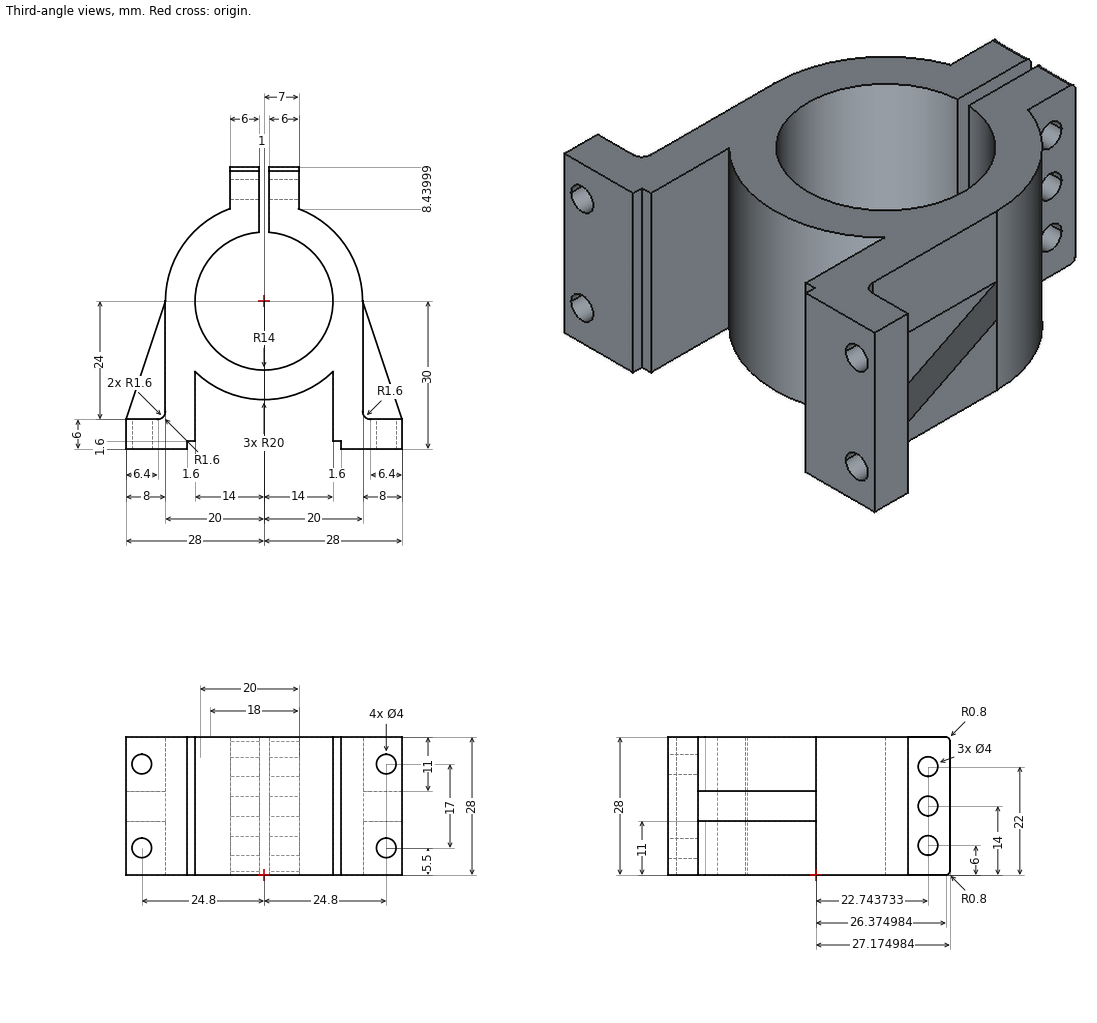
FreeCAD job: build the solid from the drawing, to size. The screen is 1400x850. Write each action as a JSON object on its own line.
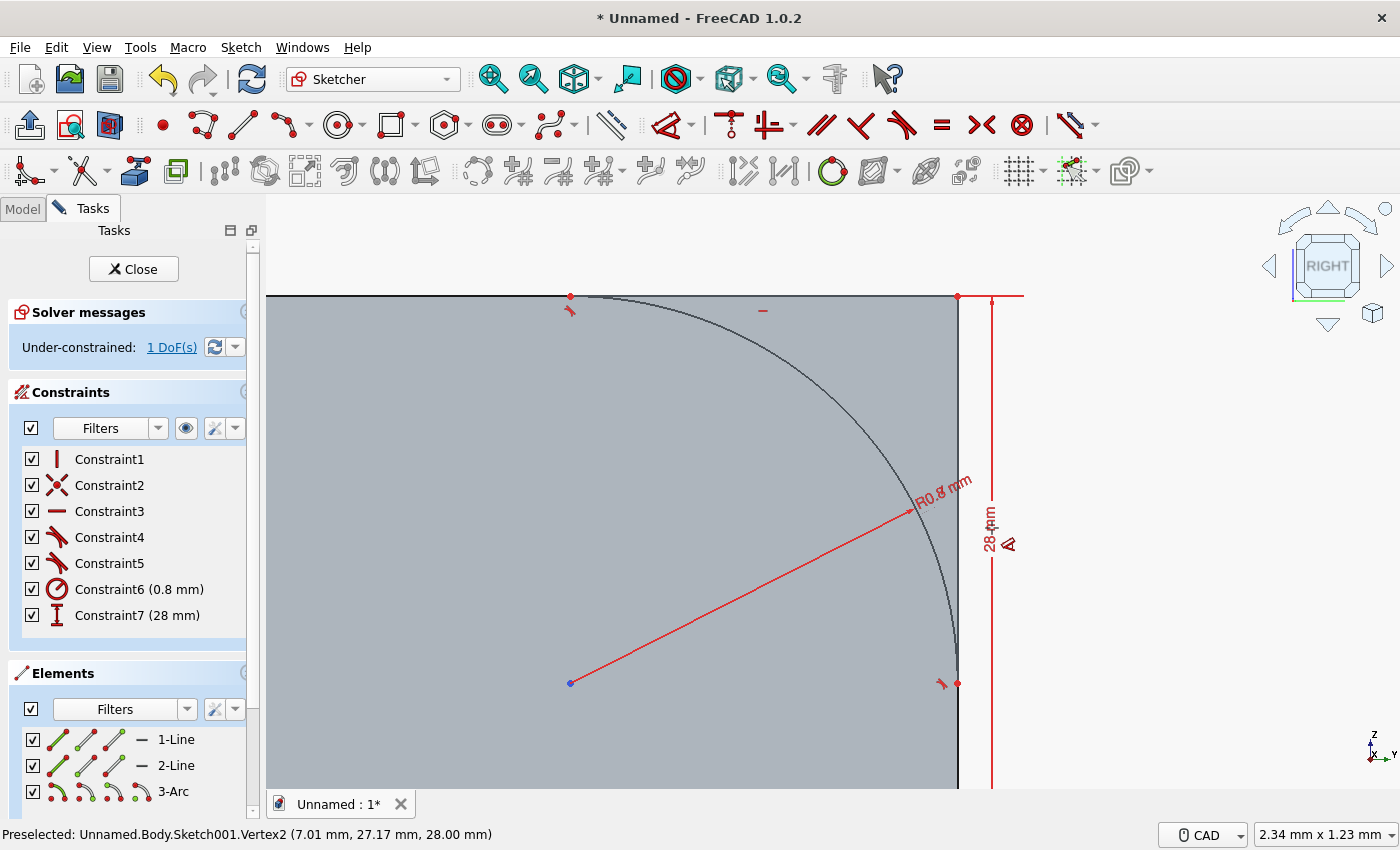
{"action": "left_click", "coordinate": [958, 684]}
{"action": "left_click", "coordinate": [626, 650]}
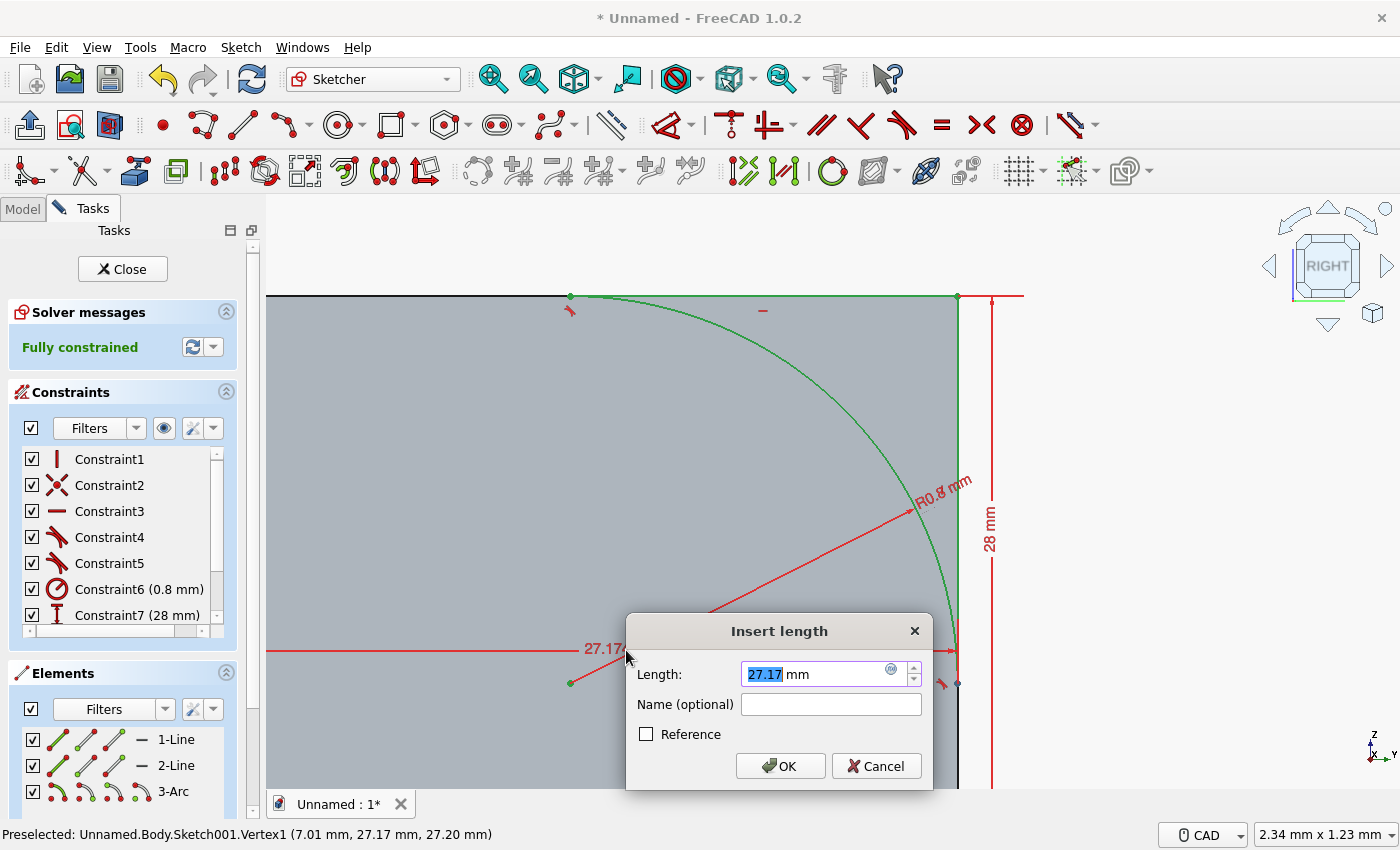
{"action": "type", "text": "27.174984"}
{"action": "key", "text": "Return"}
{"action": "key", "text": "Escape"}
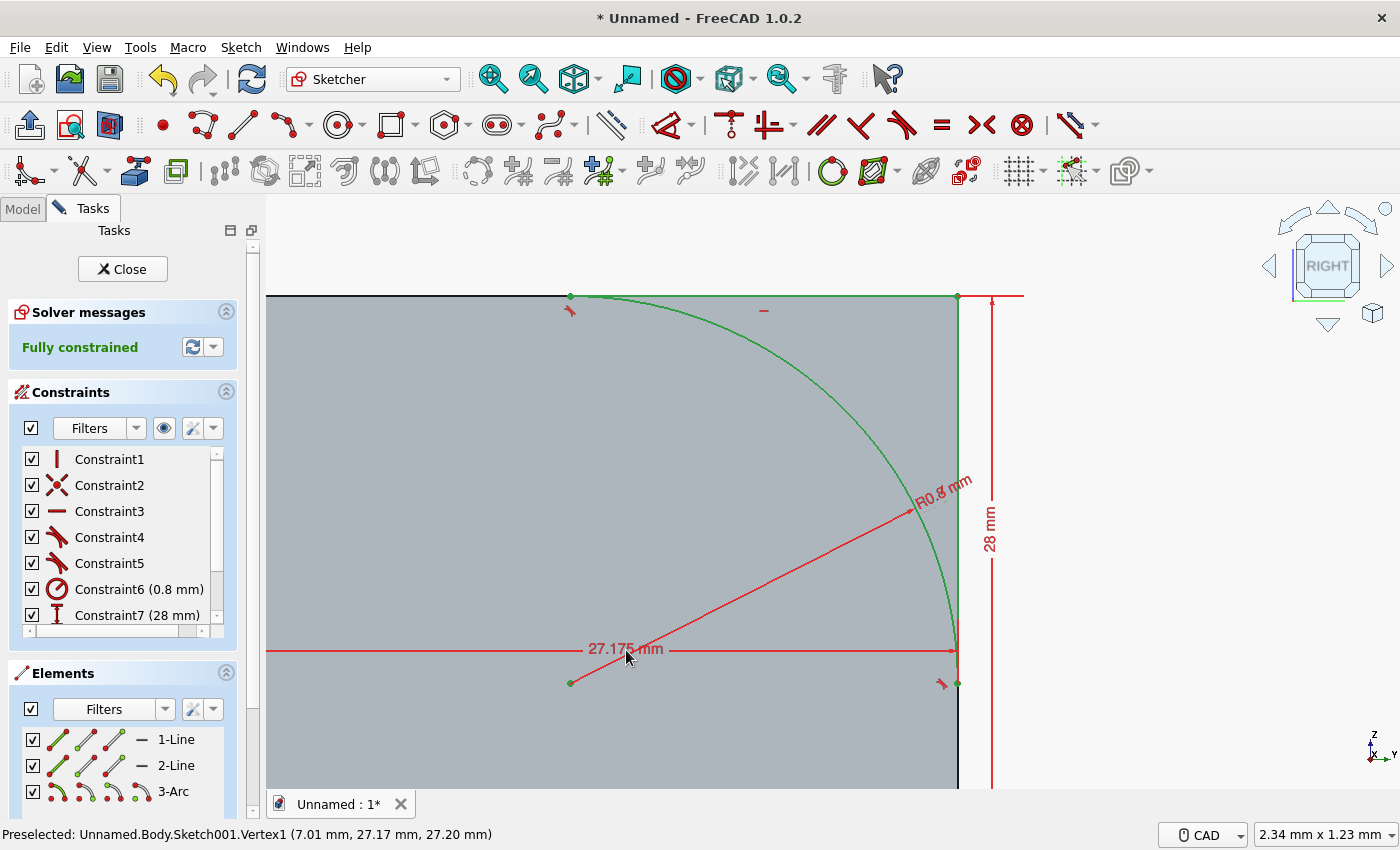
{"action": "left_click", "coordinate": [123, 269]}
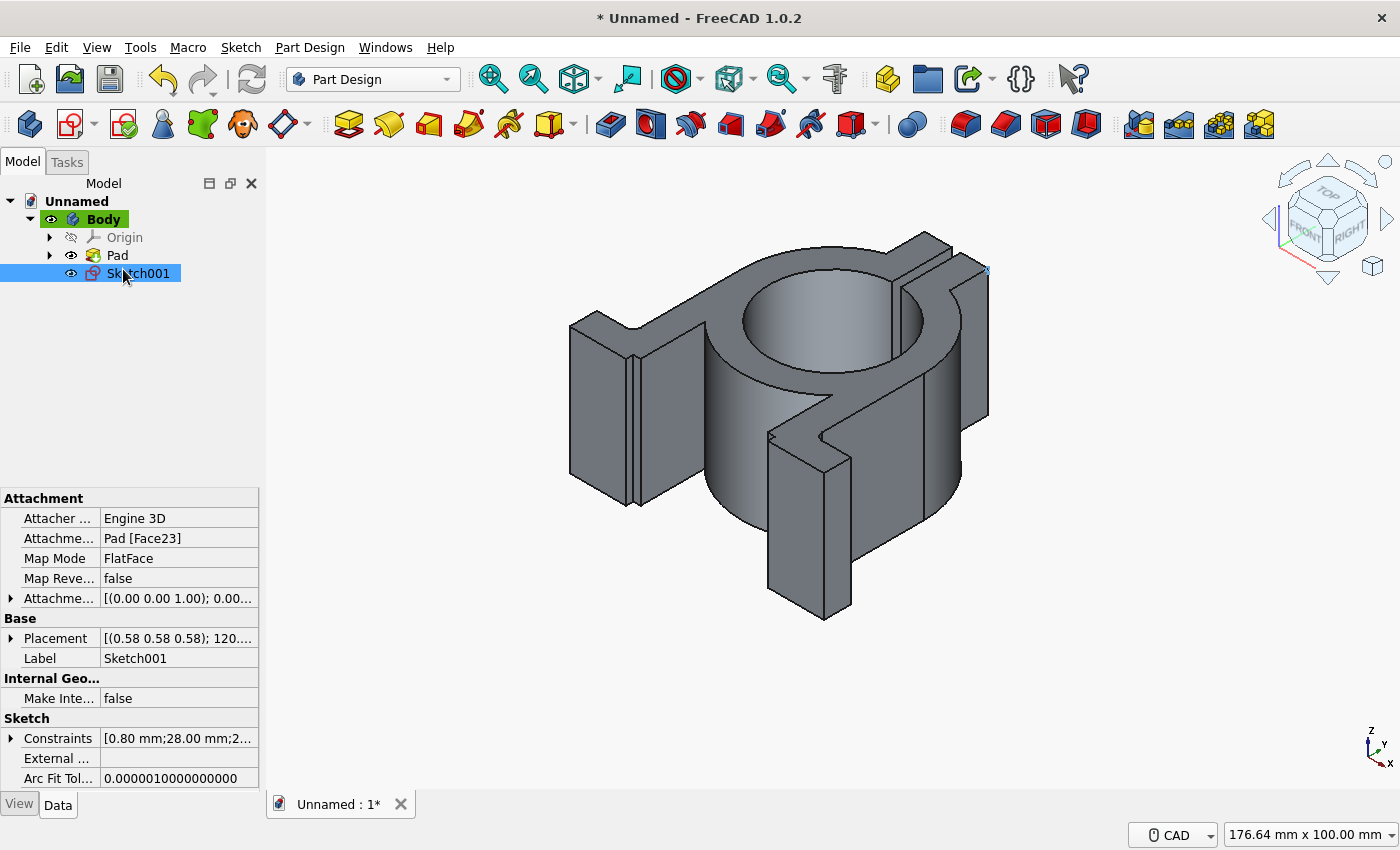
{"action": "left_click", "coordinate": [612, 124]}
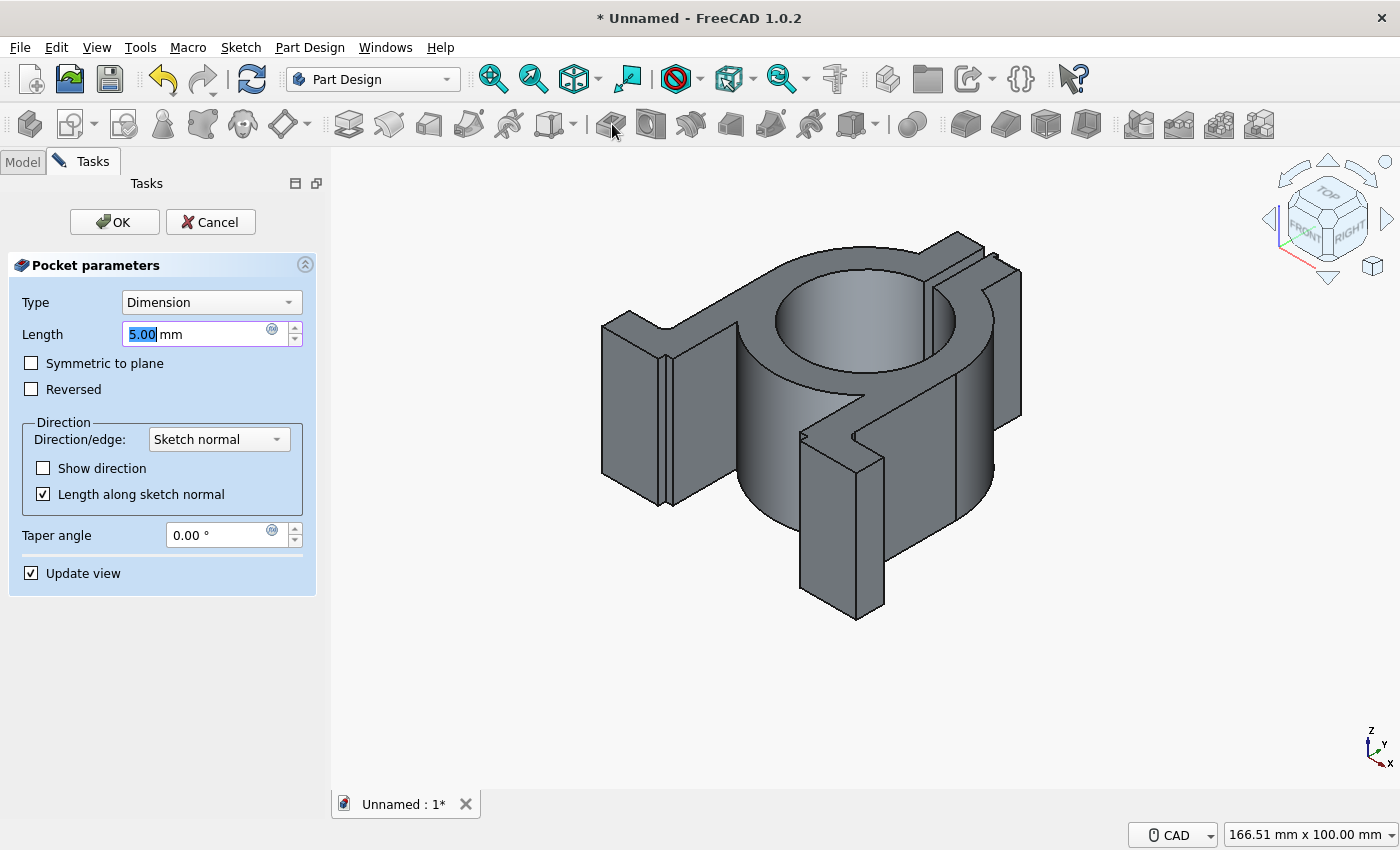
{"action": "type", "text": "18"}
{"action": "key", "text": "Tab"}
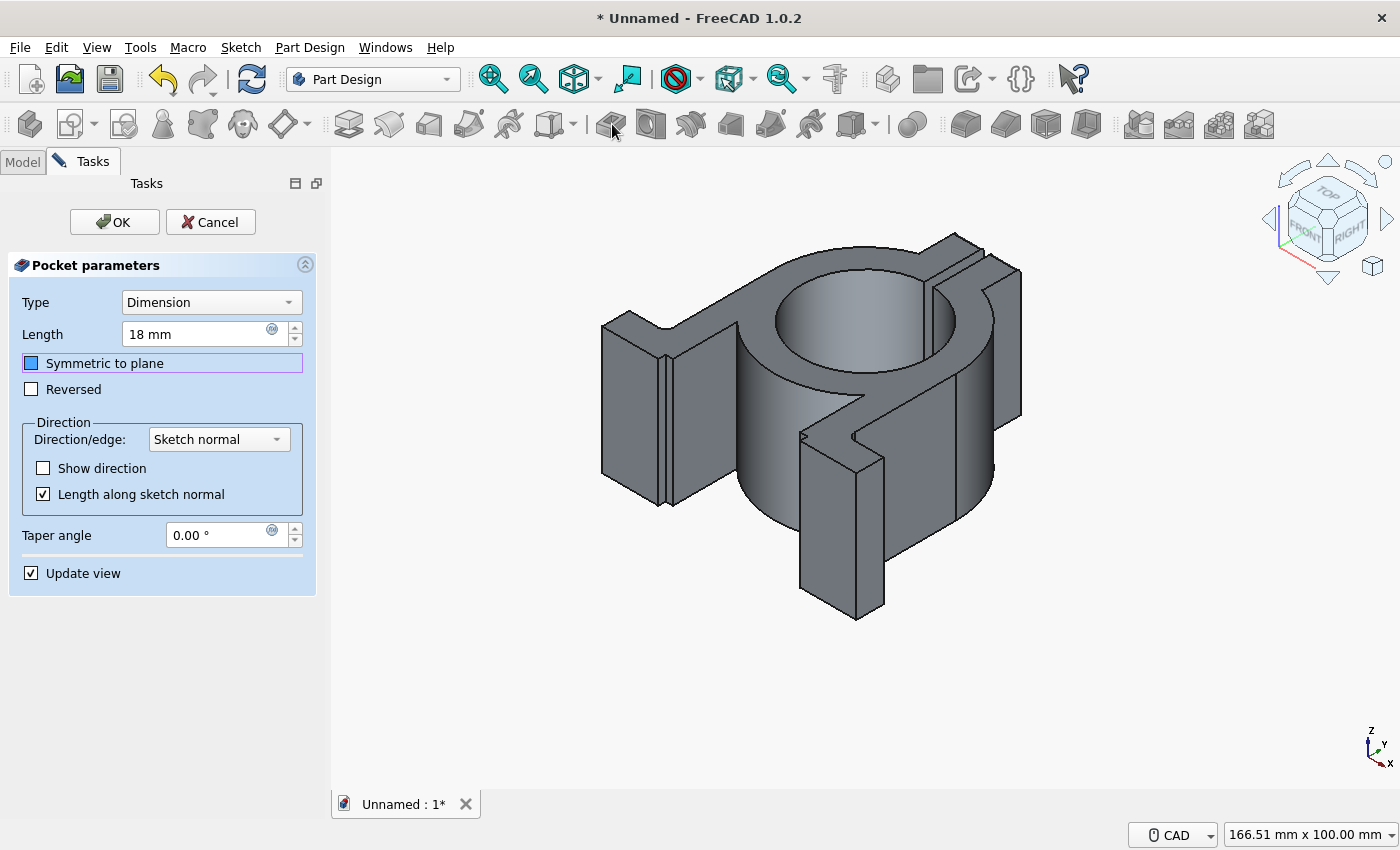
{"action": "left_click", "coordinate": [115, 222]}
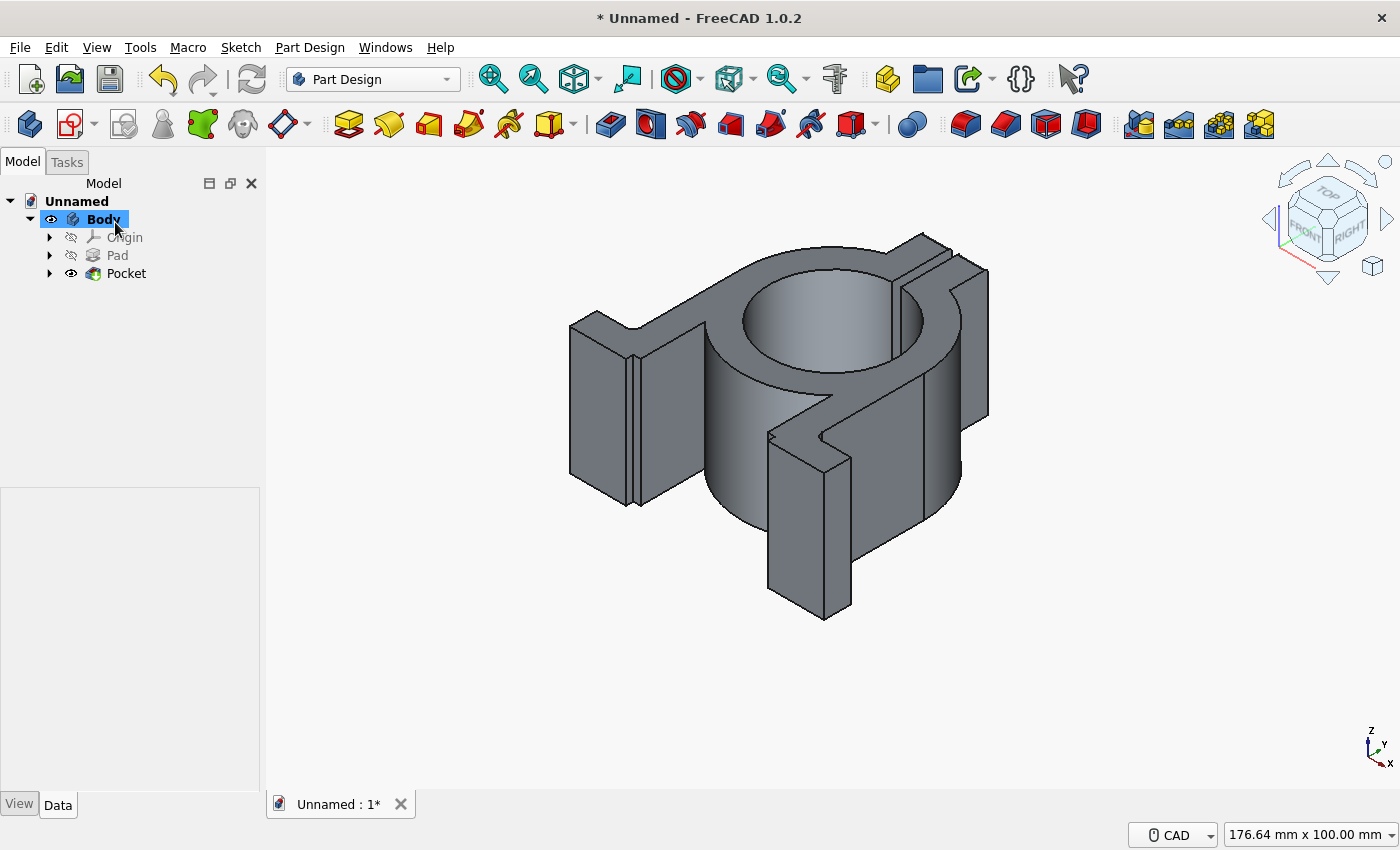
{"action": "left_click", "coordinate": [969, 310]}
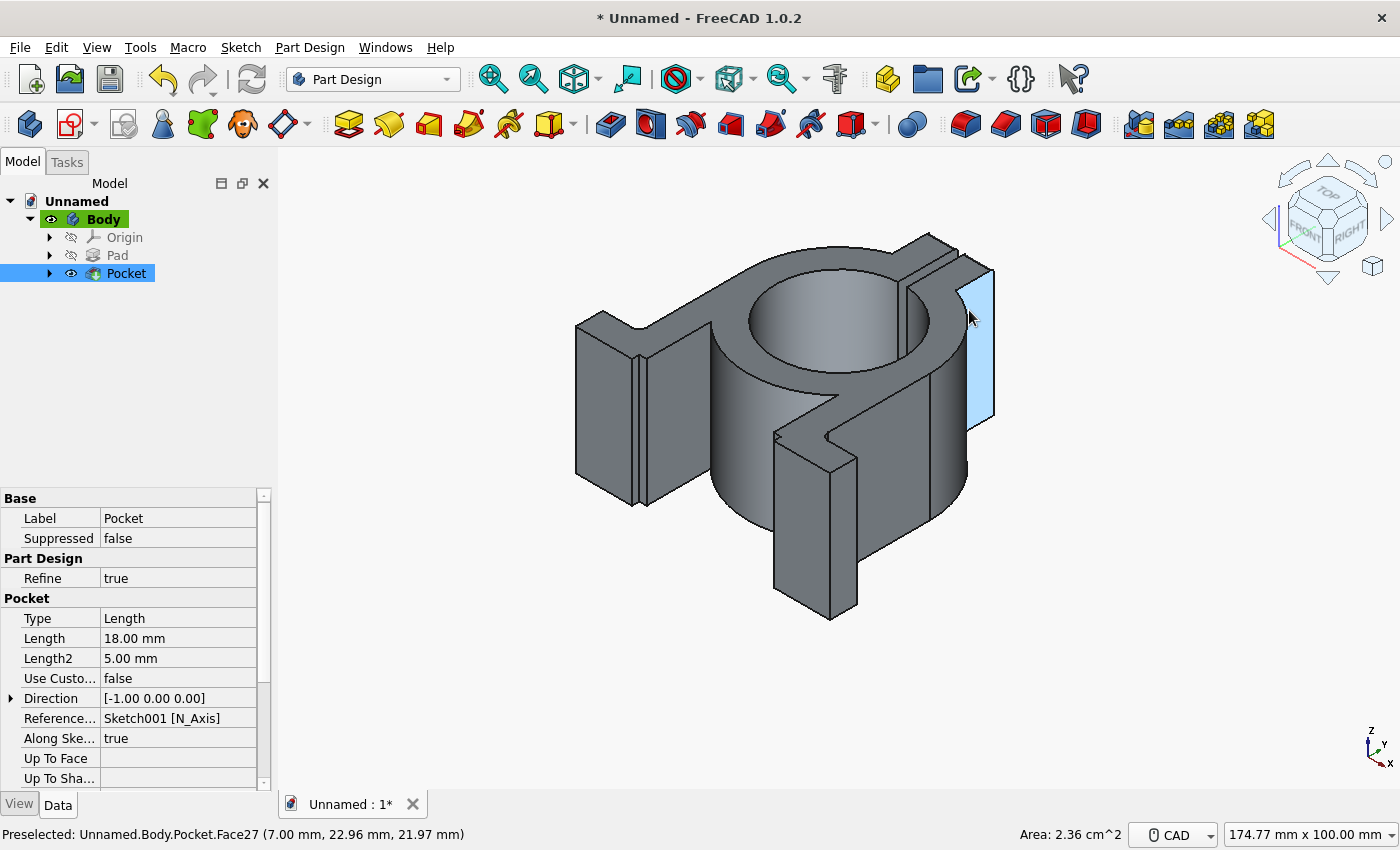
{"action": "left_click", "coordinate": [70, 124]}